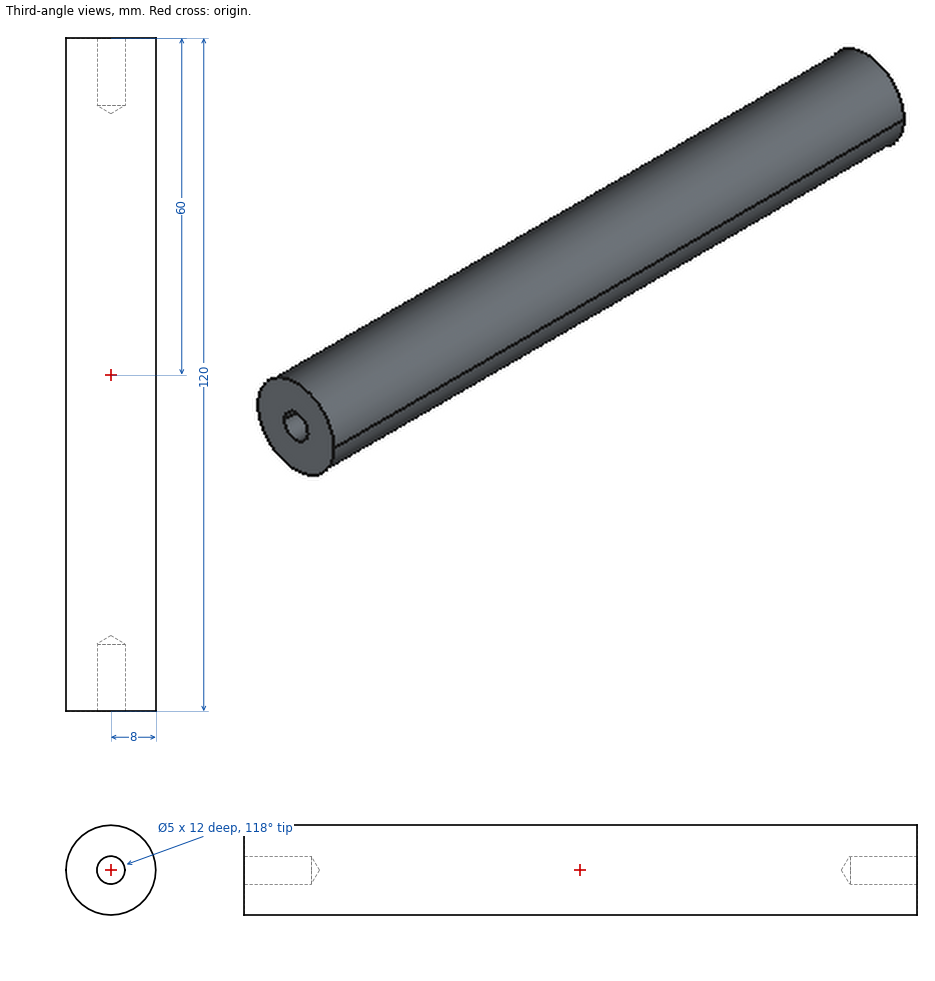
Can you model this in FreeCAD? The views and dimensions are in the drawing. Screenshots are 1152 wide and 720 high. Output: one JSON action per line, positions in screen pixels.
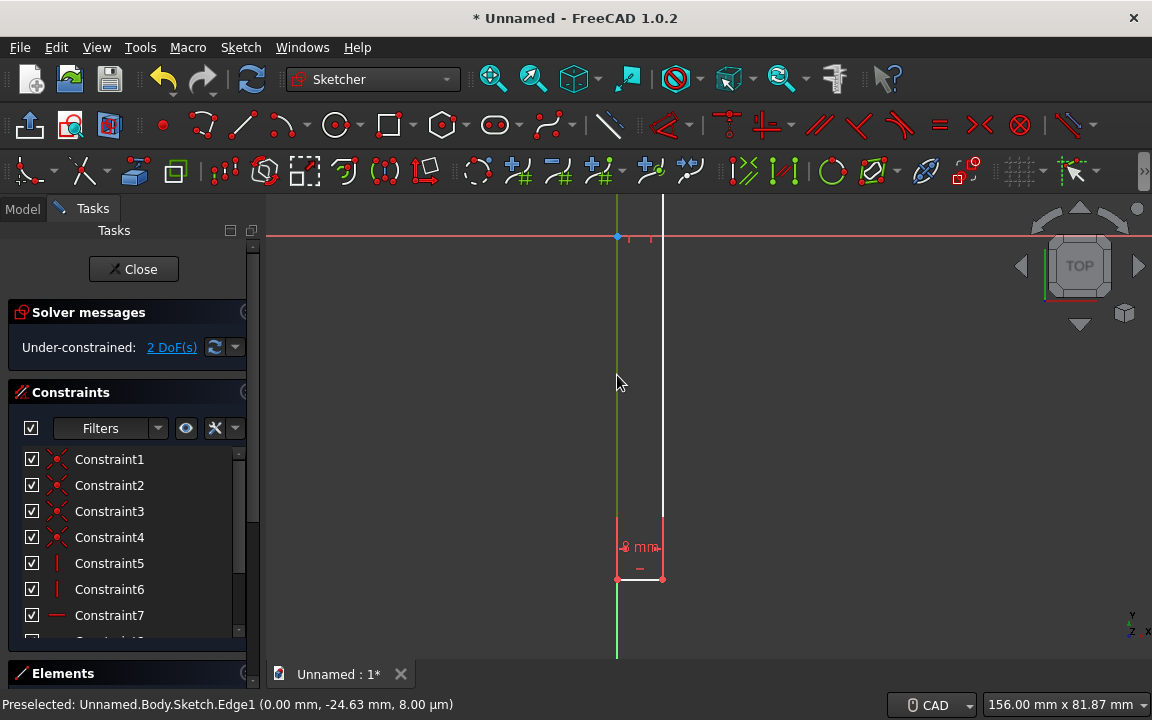
{"action": "key", "text": "i"}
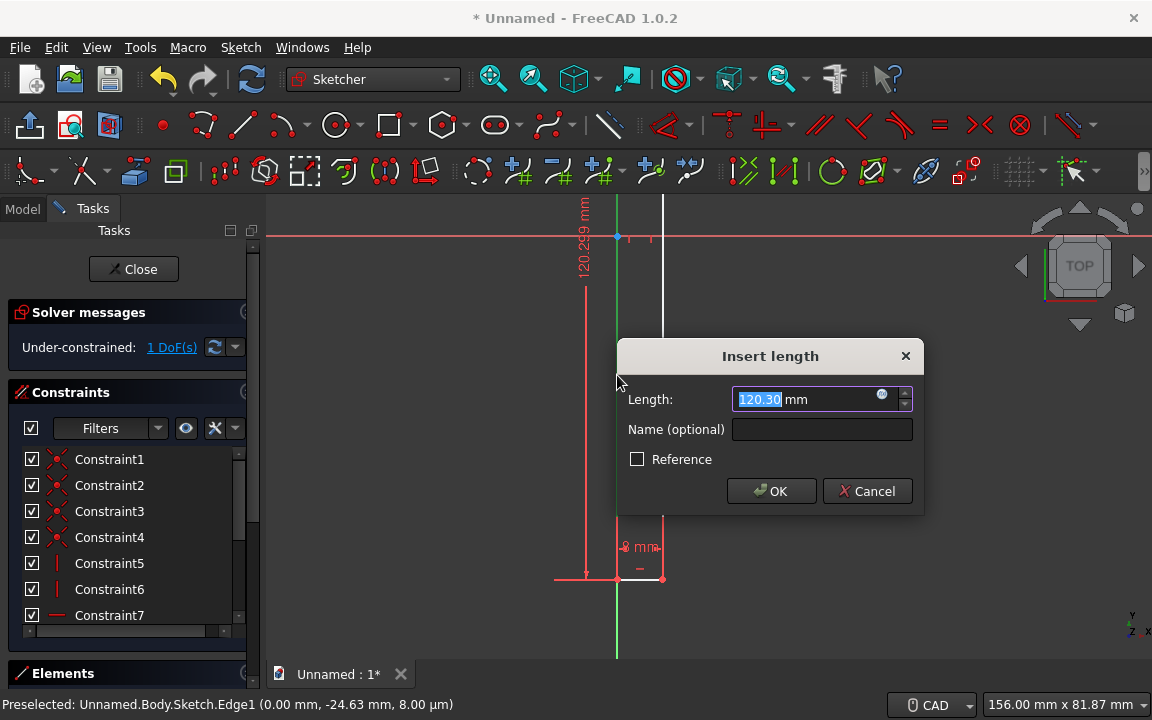
{"action": "type", "text": "120"}
{"action": "key", "text": "Return"}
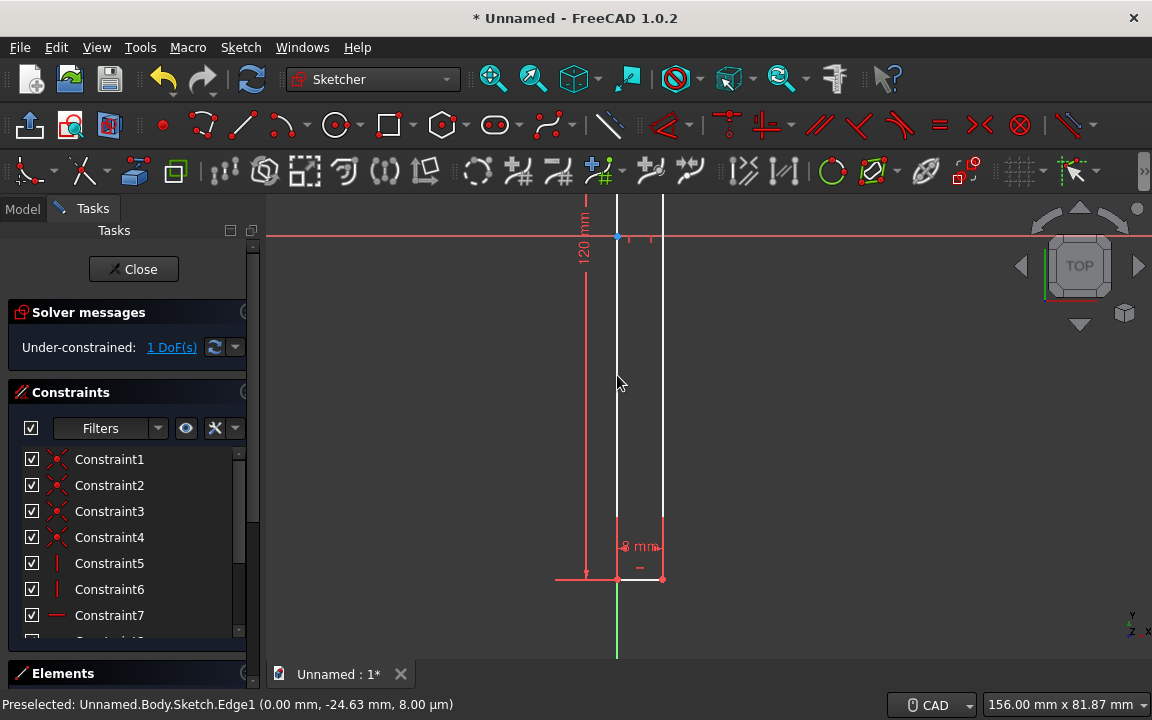
{"action": "scroll", "coordinate": [641, 582], "scroll_direction": "down", "scroll_amount": 4}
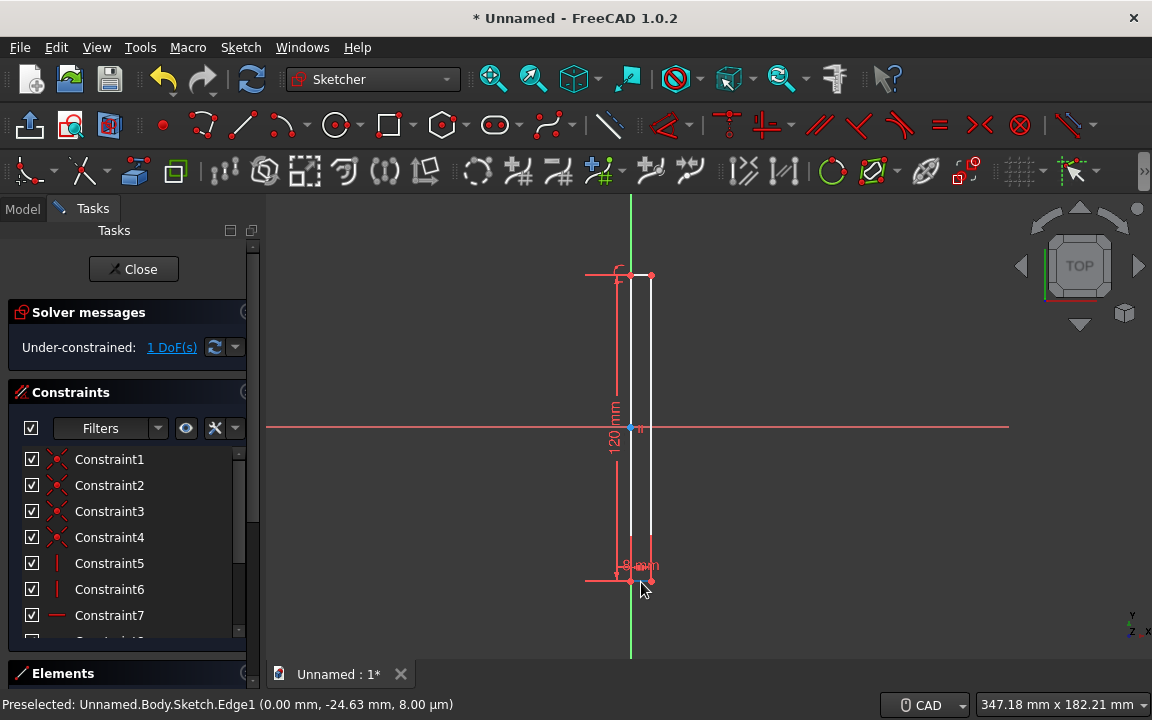
{"action": "left_click", "coordinate": [631, 275]}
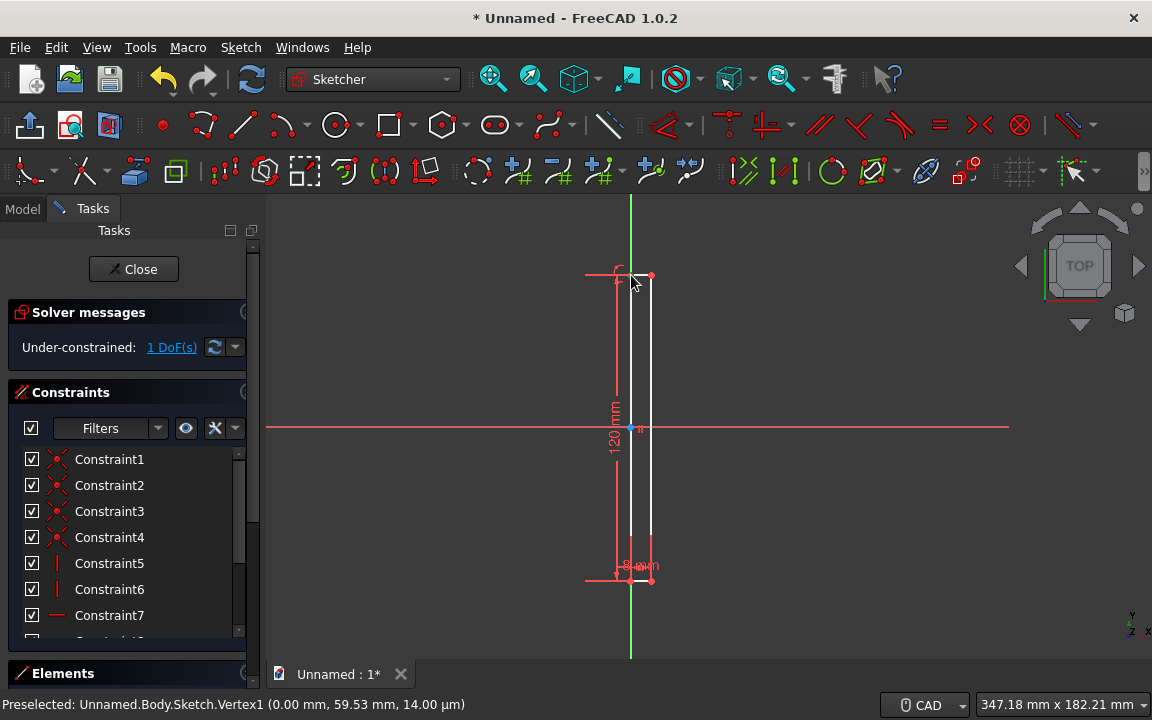
{"action": "key", "text": "i"}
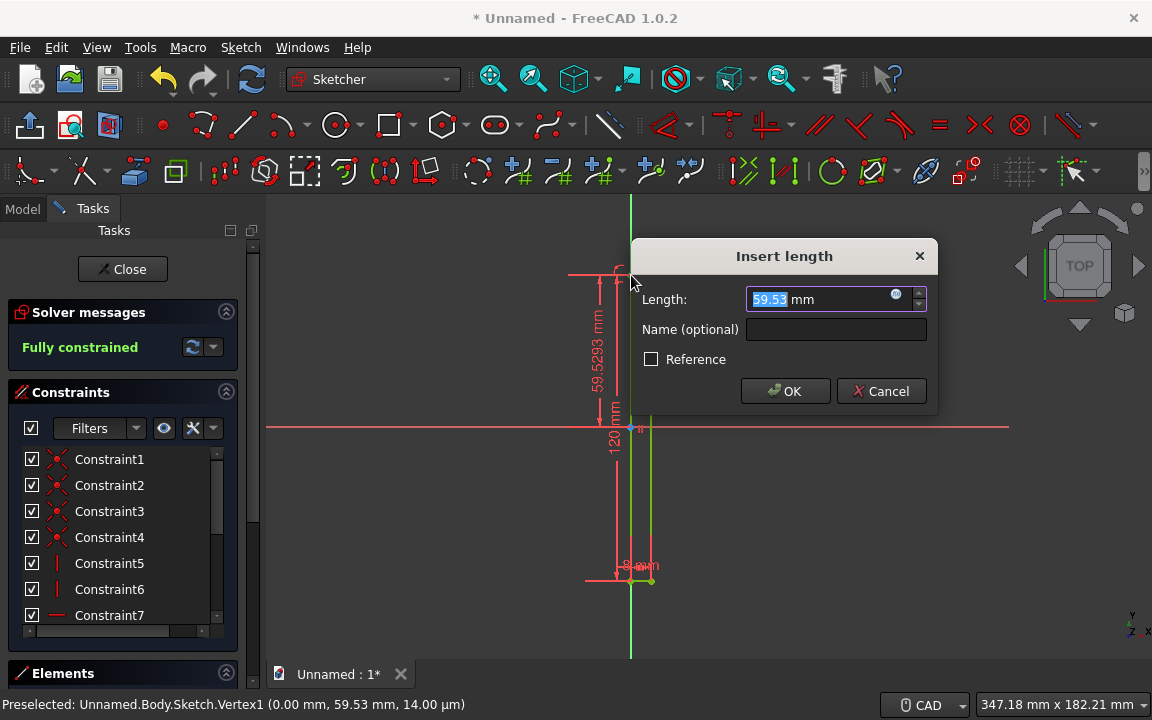
{"action": "type", "text": "60"}
{"action": "key", "text": "Return"}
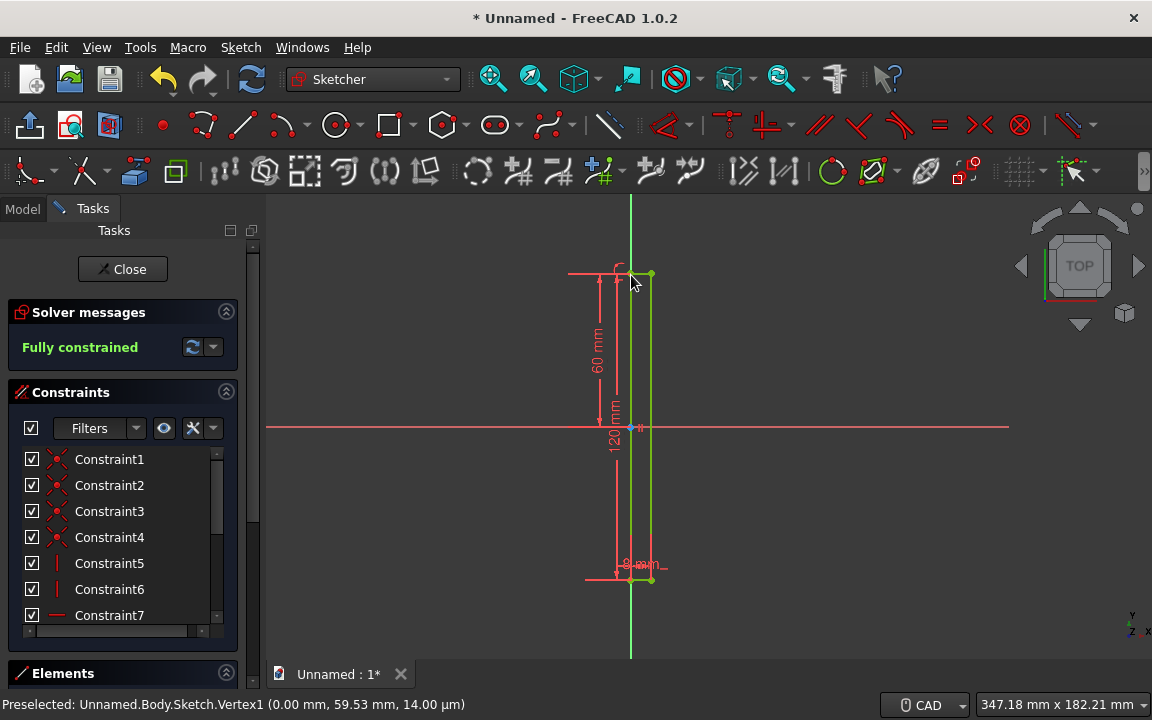
{"action": "left_click", "coordinate": [123, 269]}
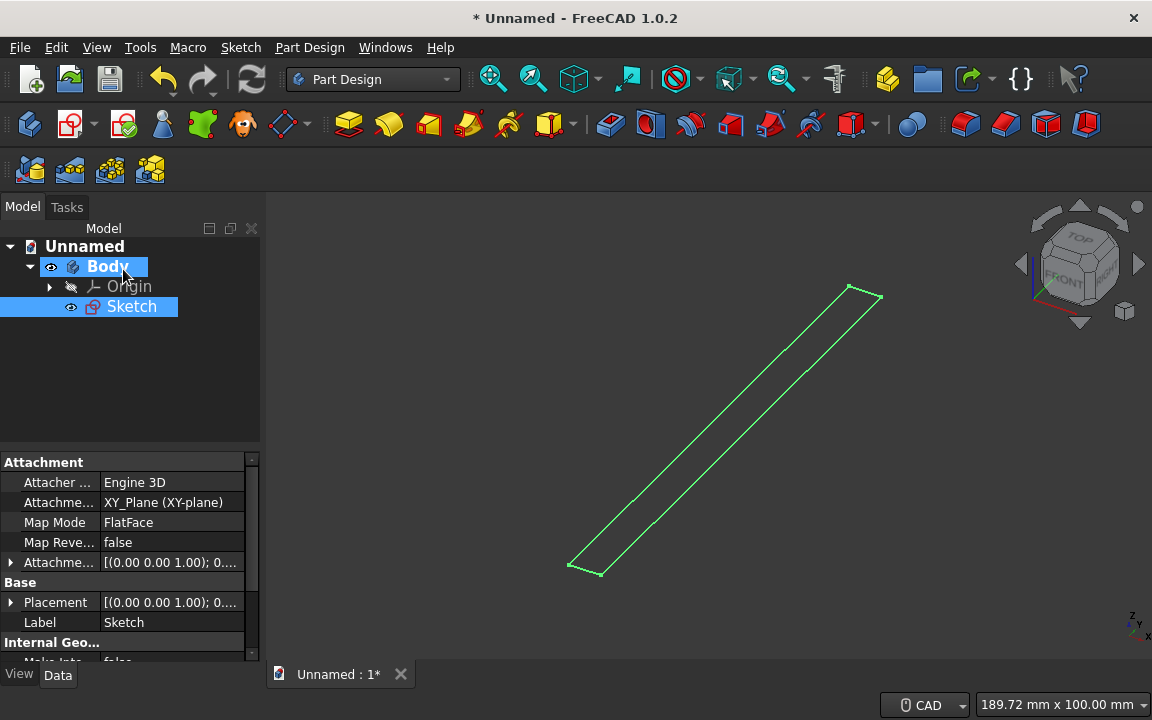
{"action": "left_click", "coordinate": [390, 124]}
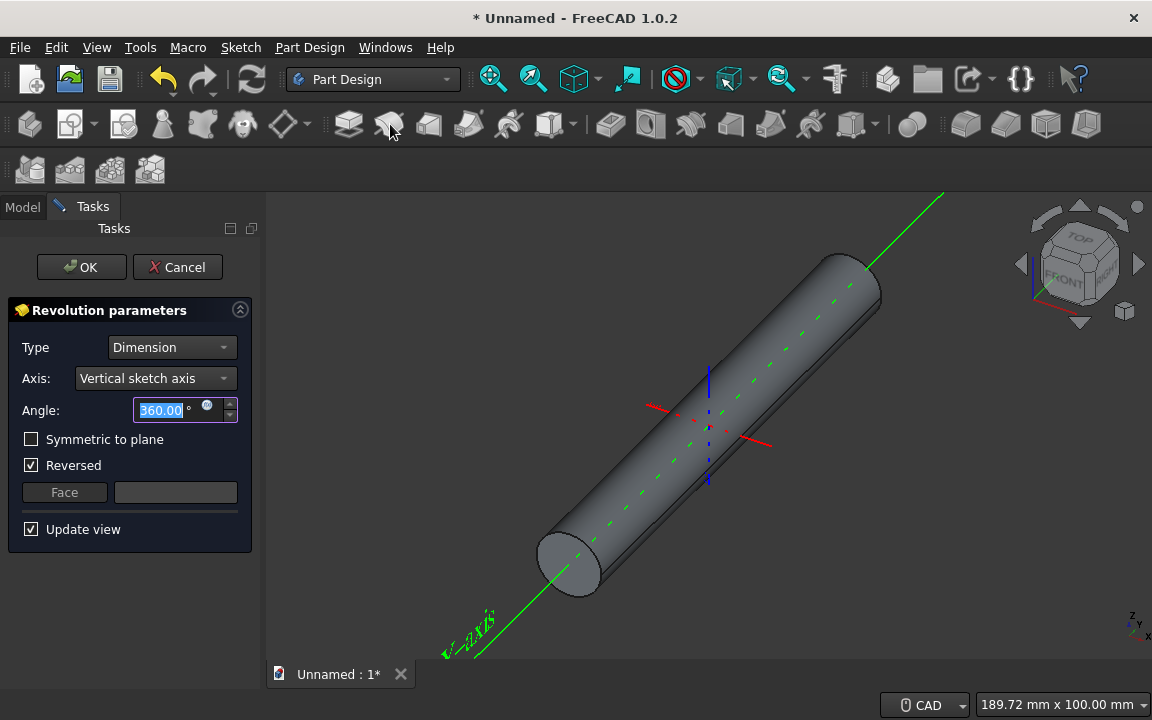
{"action": "left_click", "coordinate": [82, 267]}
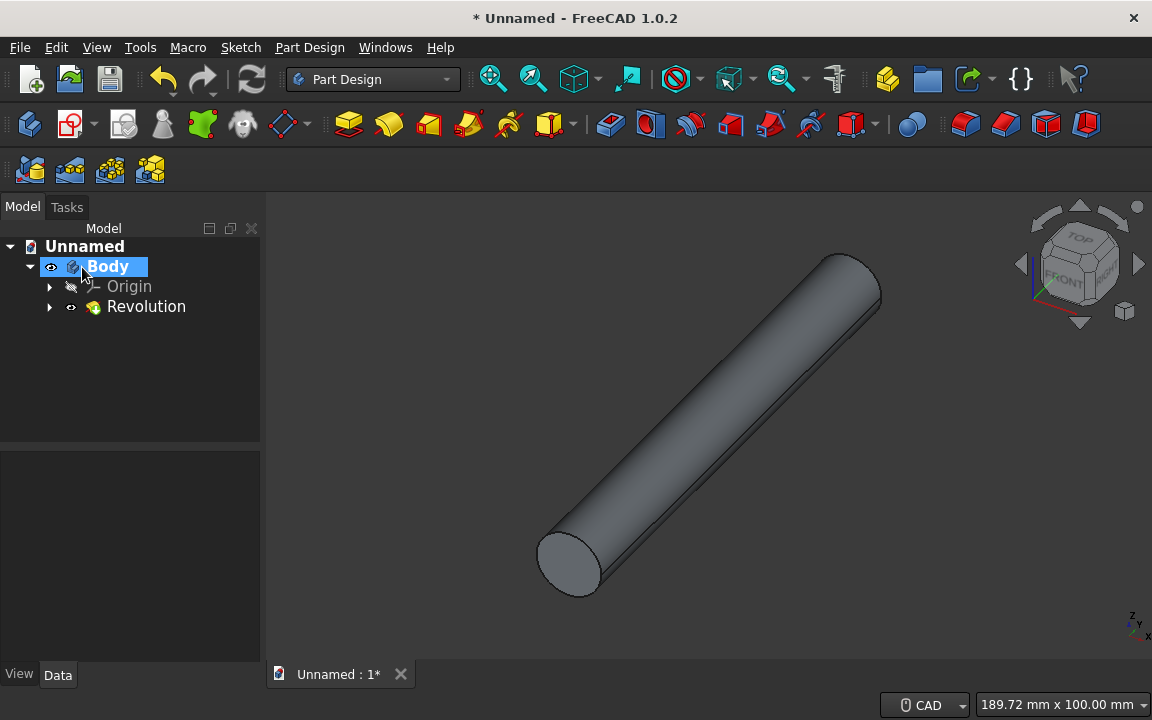
{"action": "key", "text": "4"}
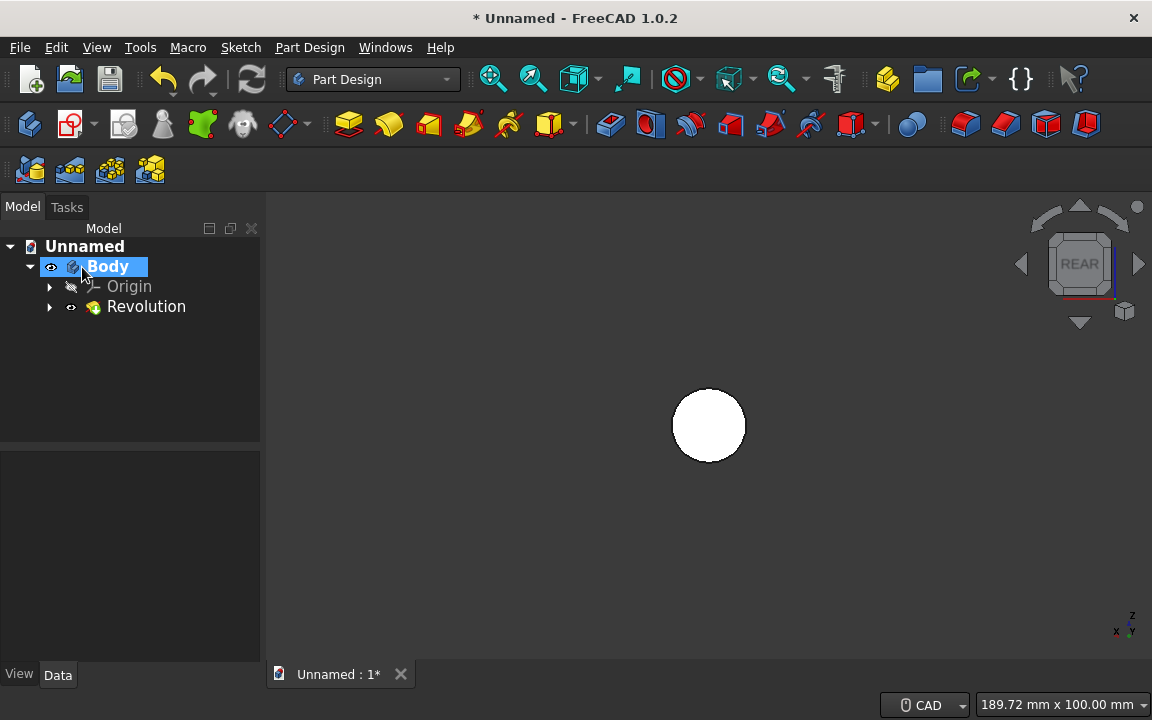
{"action": "key", "text": "v f"}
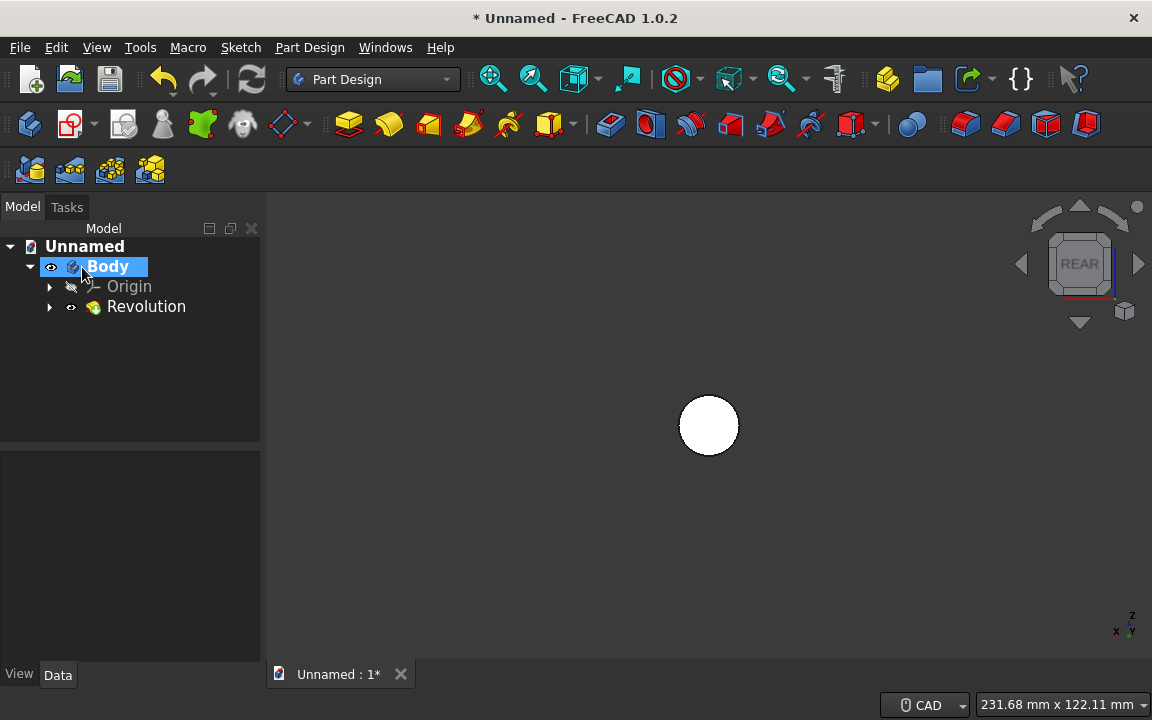
{"action": "left_click", "coordinate": [709, 425]}